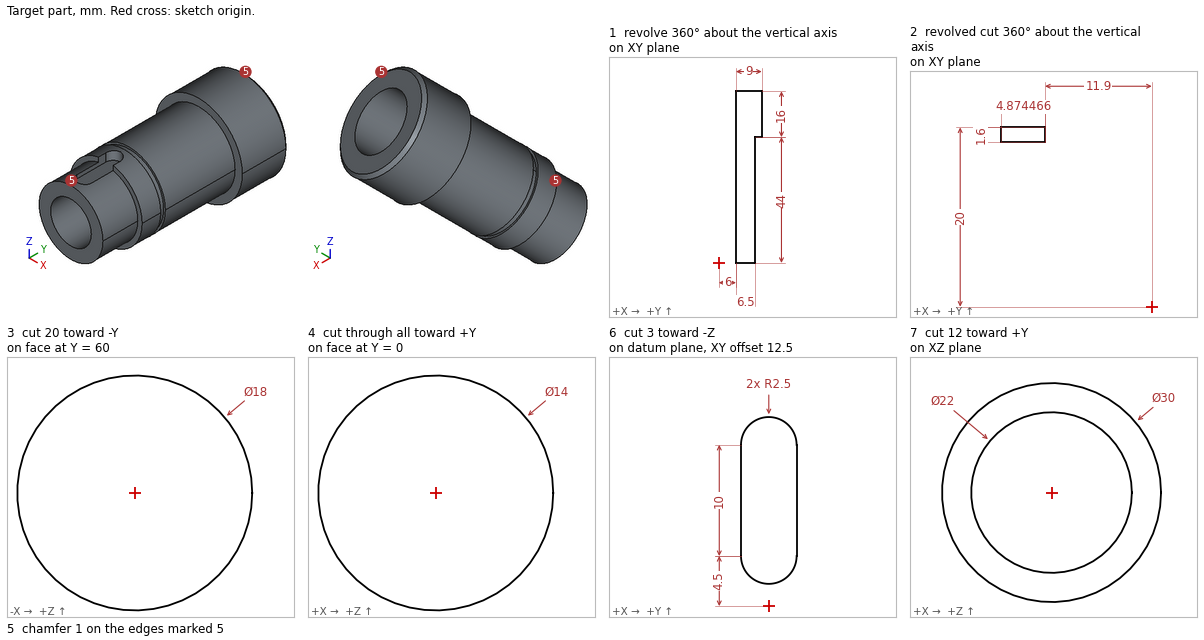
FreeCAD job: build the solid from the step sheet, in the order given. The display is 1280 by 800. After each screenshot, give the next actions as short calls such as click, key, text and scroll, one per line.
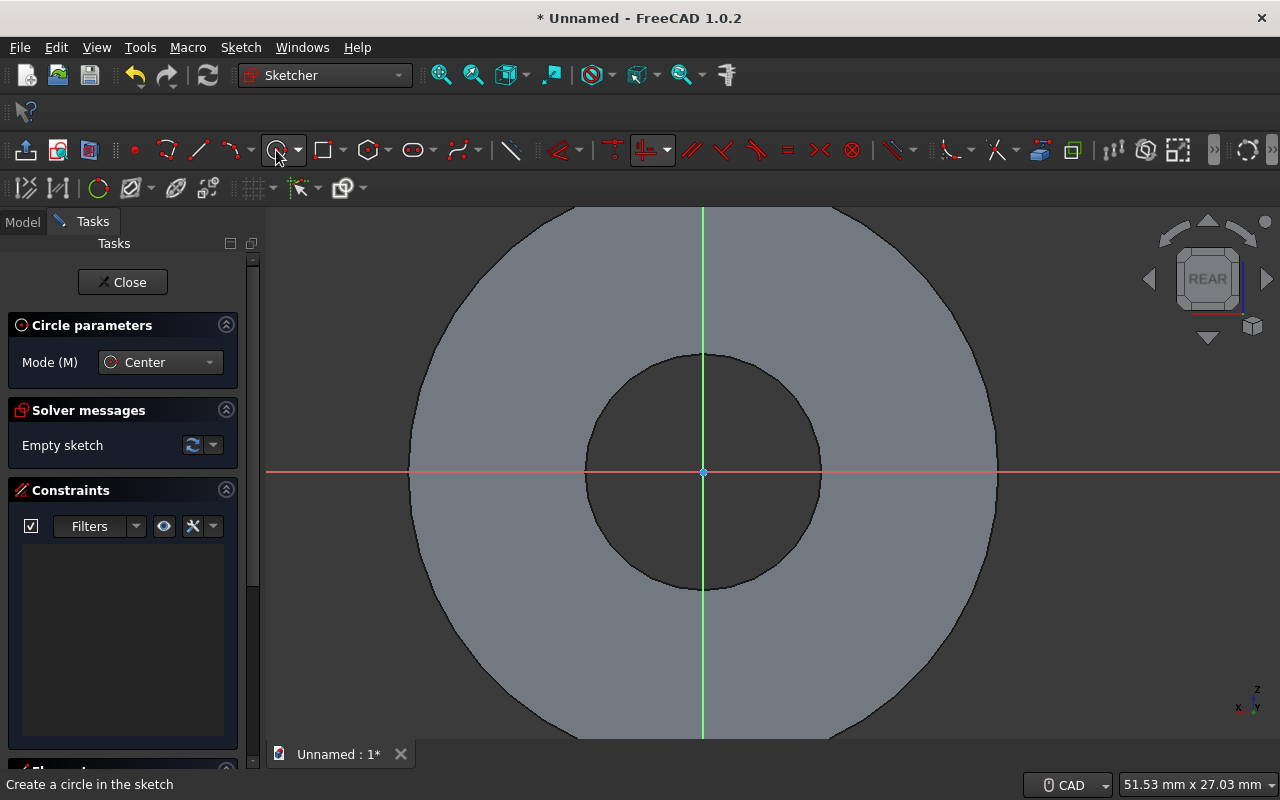
click(703, 472)
move(829, 347)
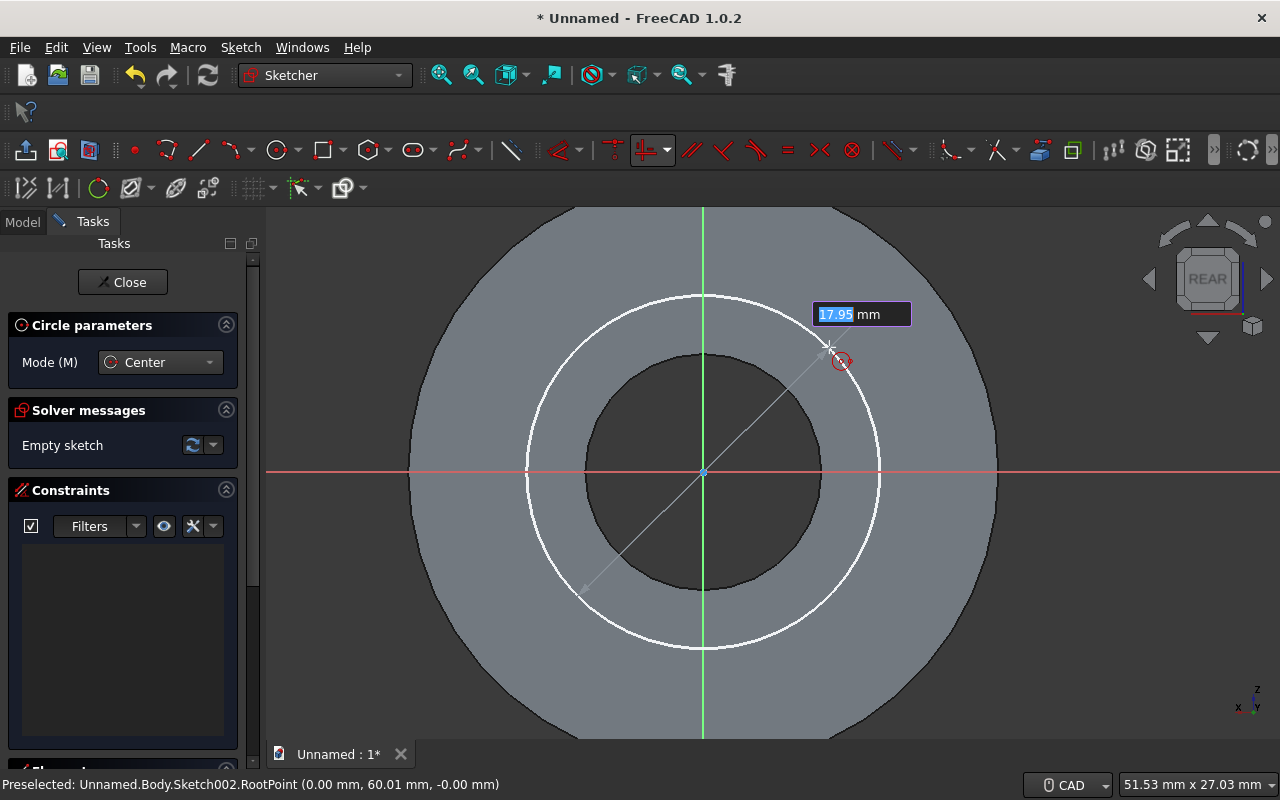
text(18)
key(Return)
key(Escape)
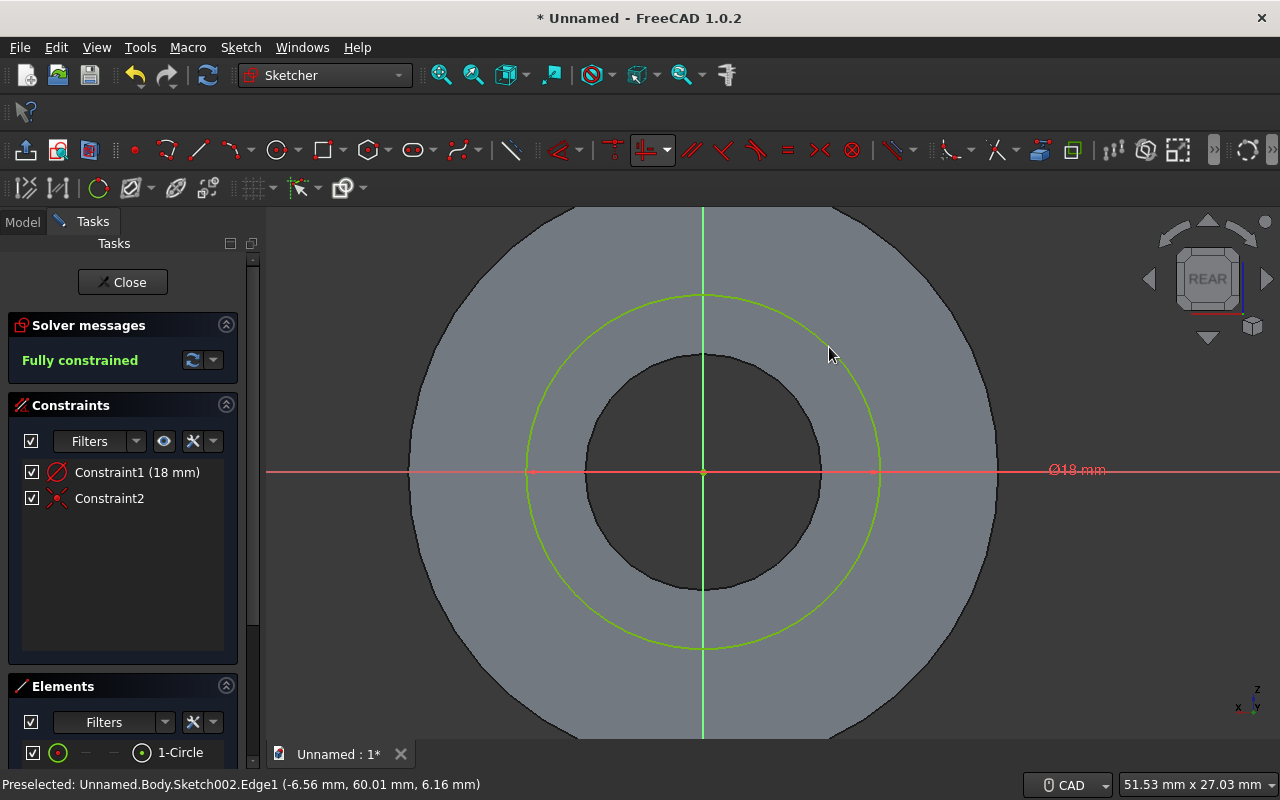
click(123, 282)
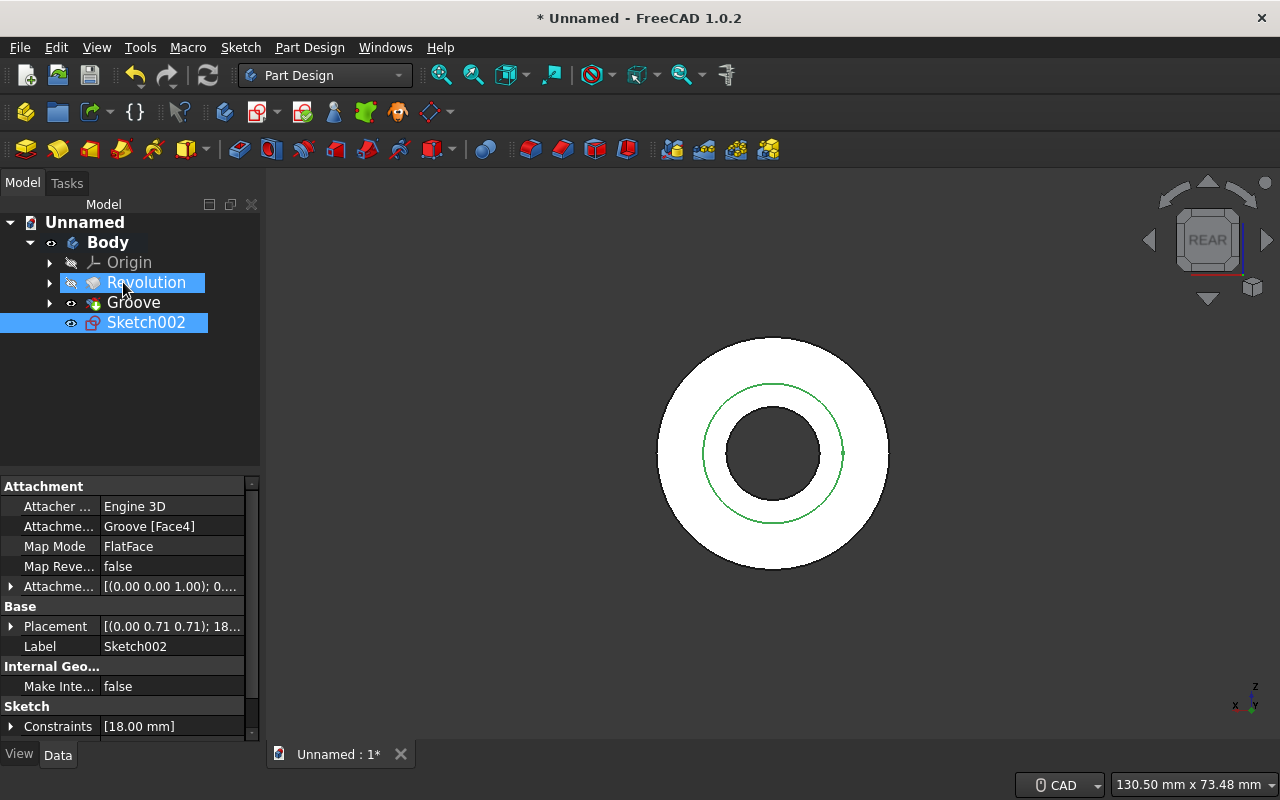
click(240, 150)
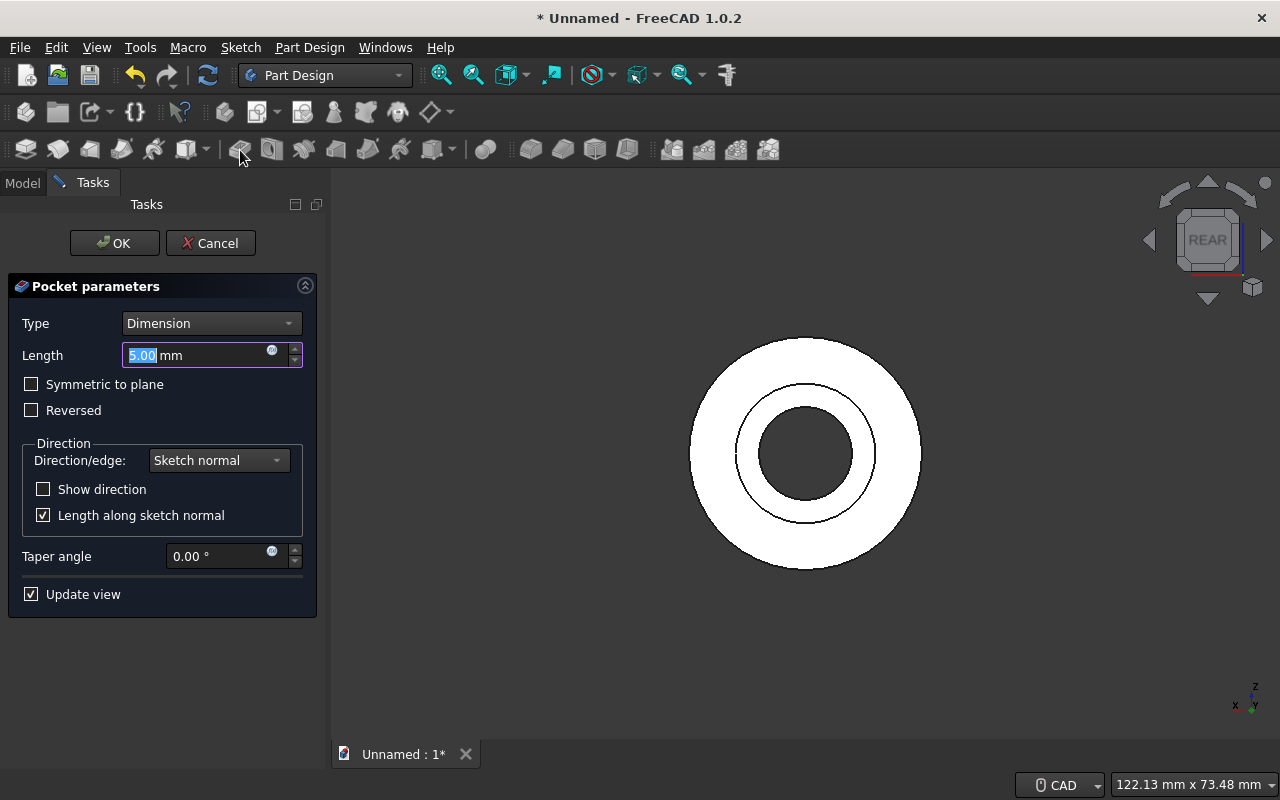
text(20)
key(Tab)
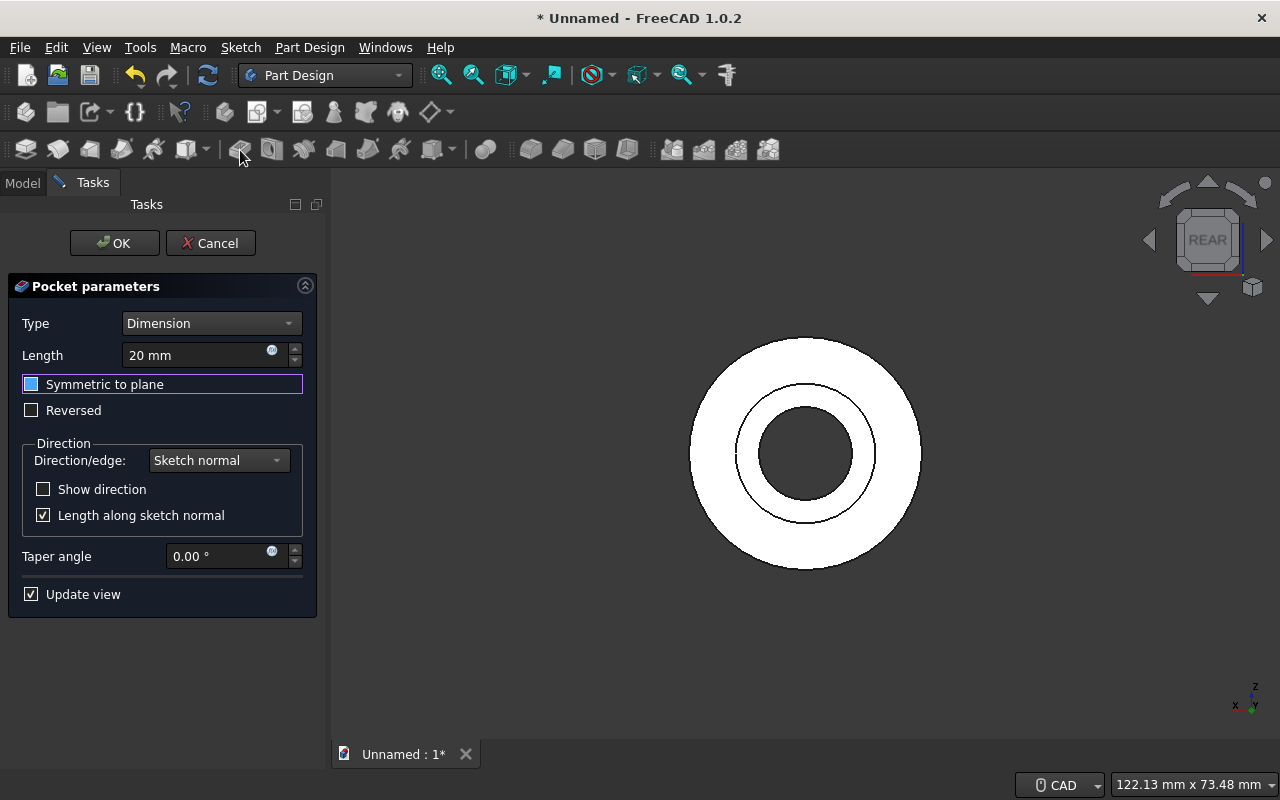
click(115, 243)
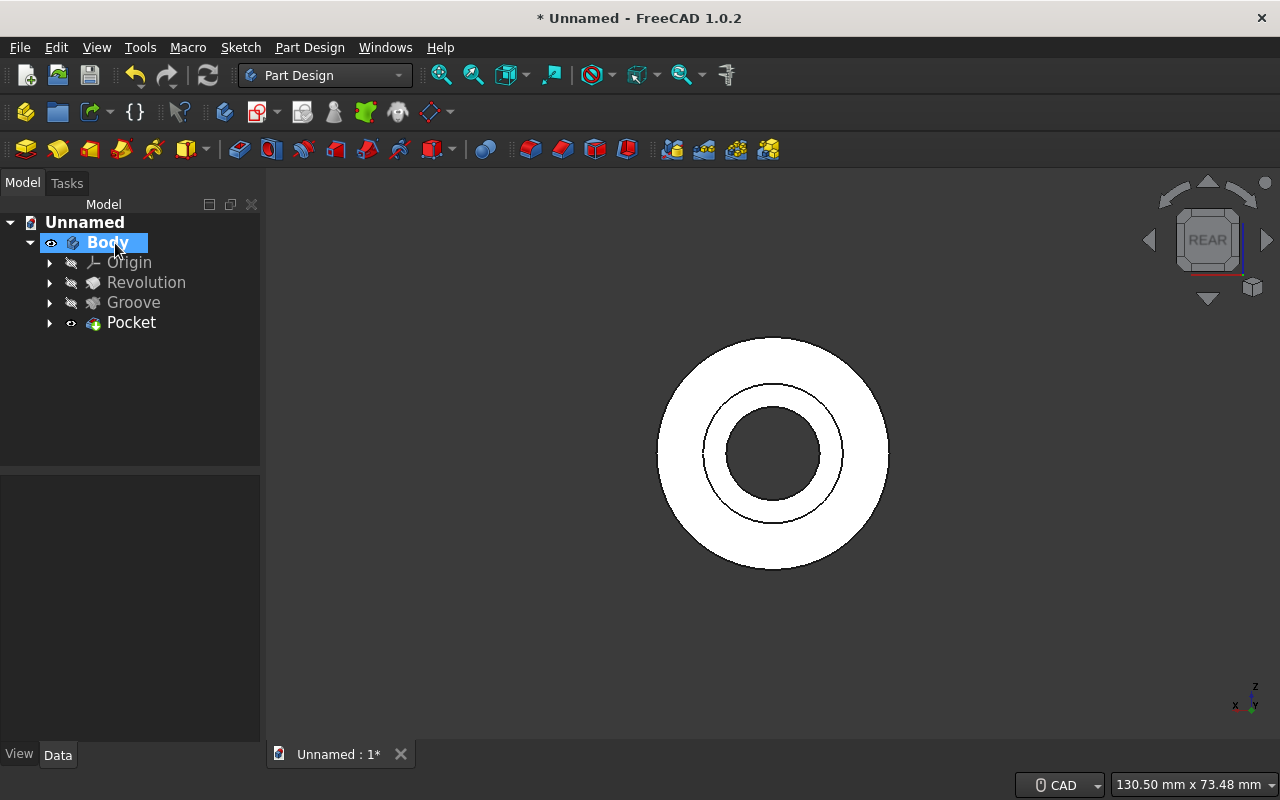
click(442, 76)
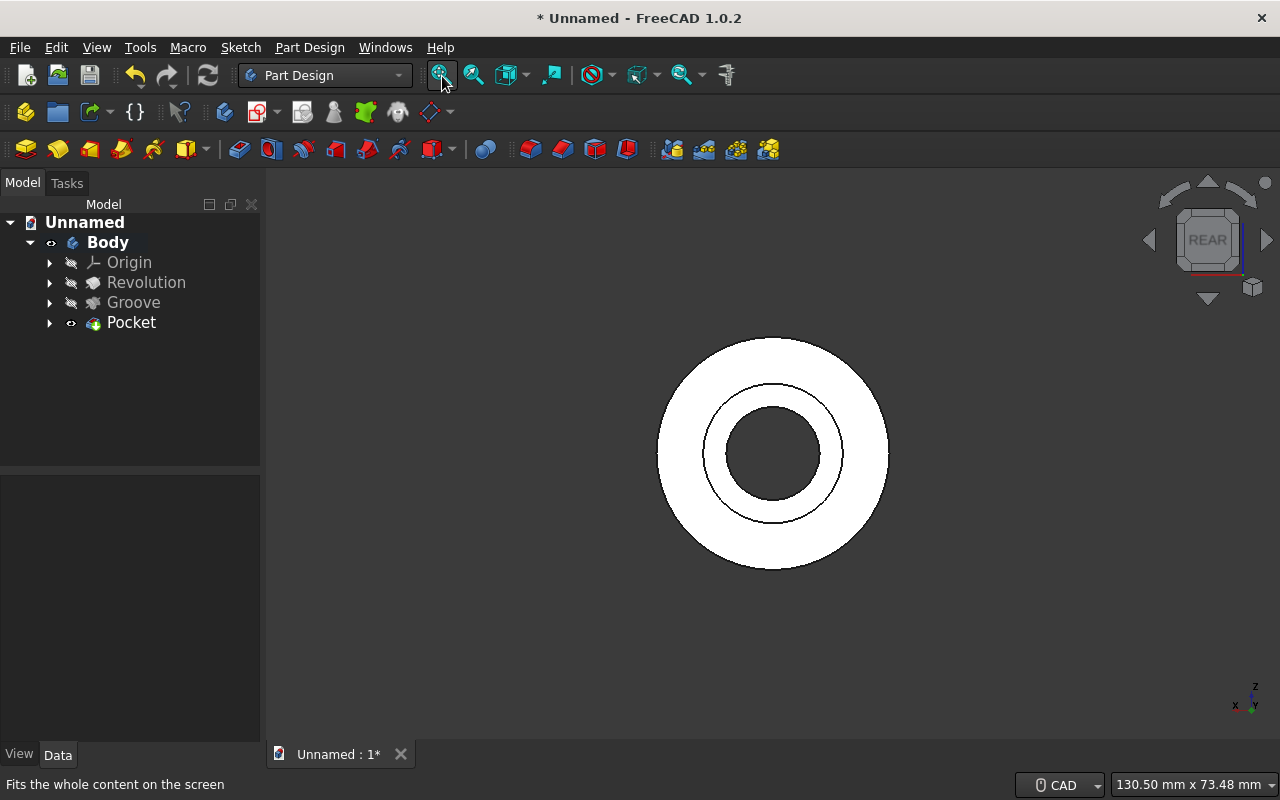
key(0)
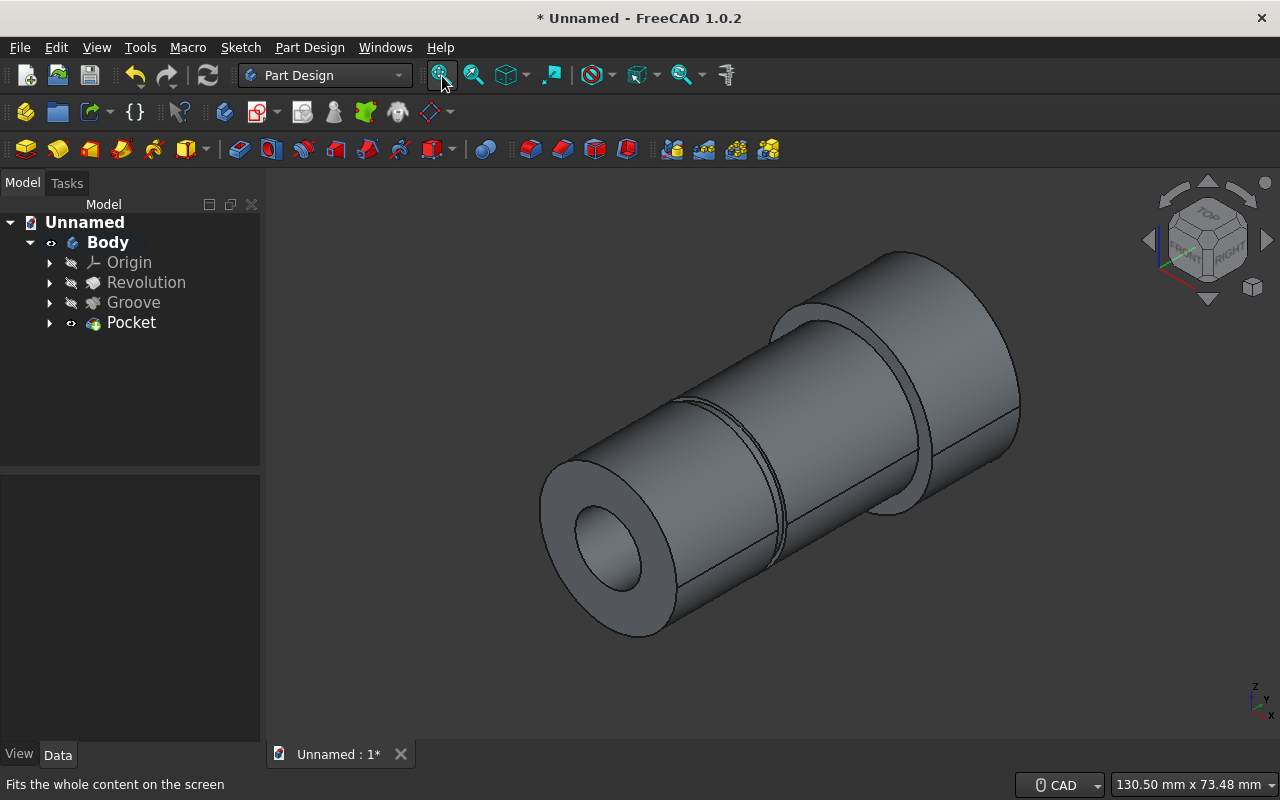
click(569, 570)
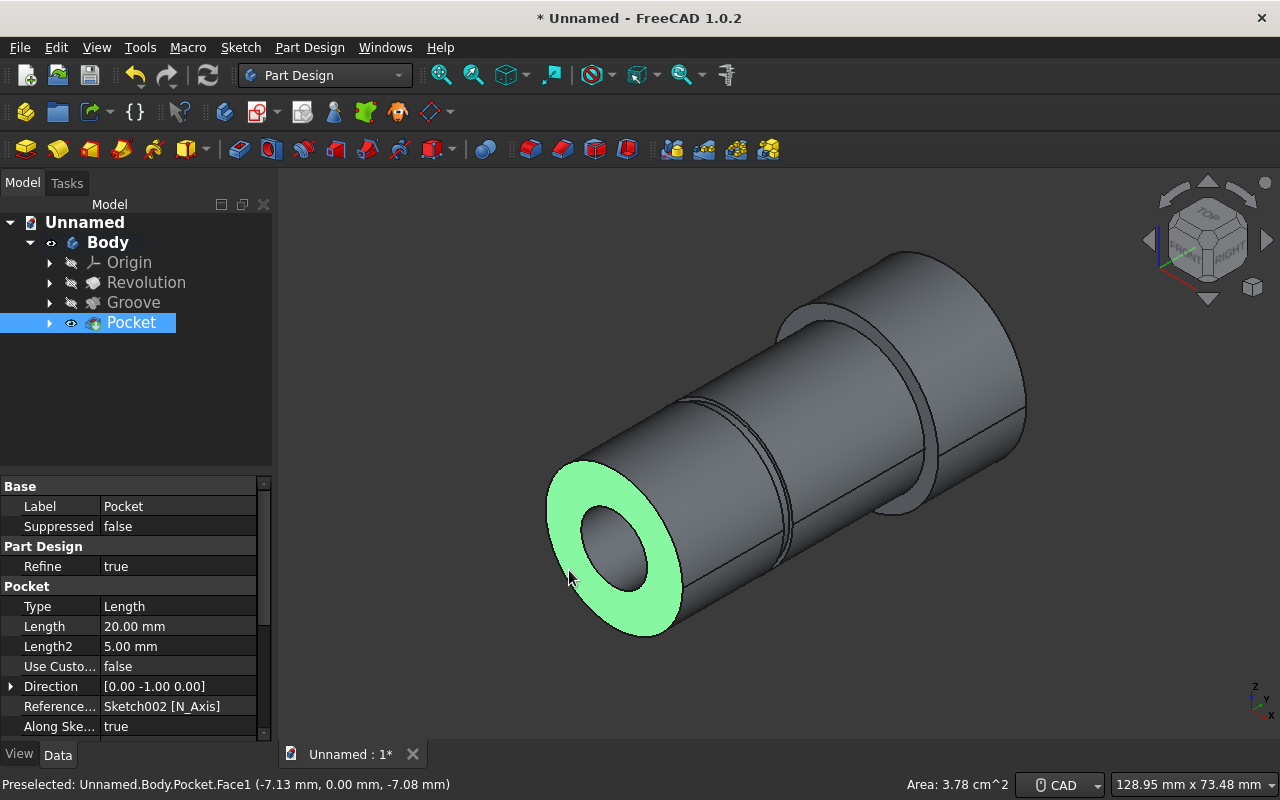
click(258, 112)